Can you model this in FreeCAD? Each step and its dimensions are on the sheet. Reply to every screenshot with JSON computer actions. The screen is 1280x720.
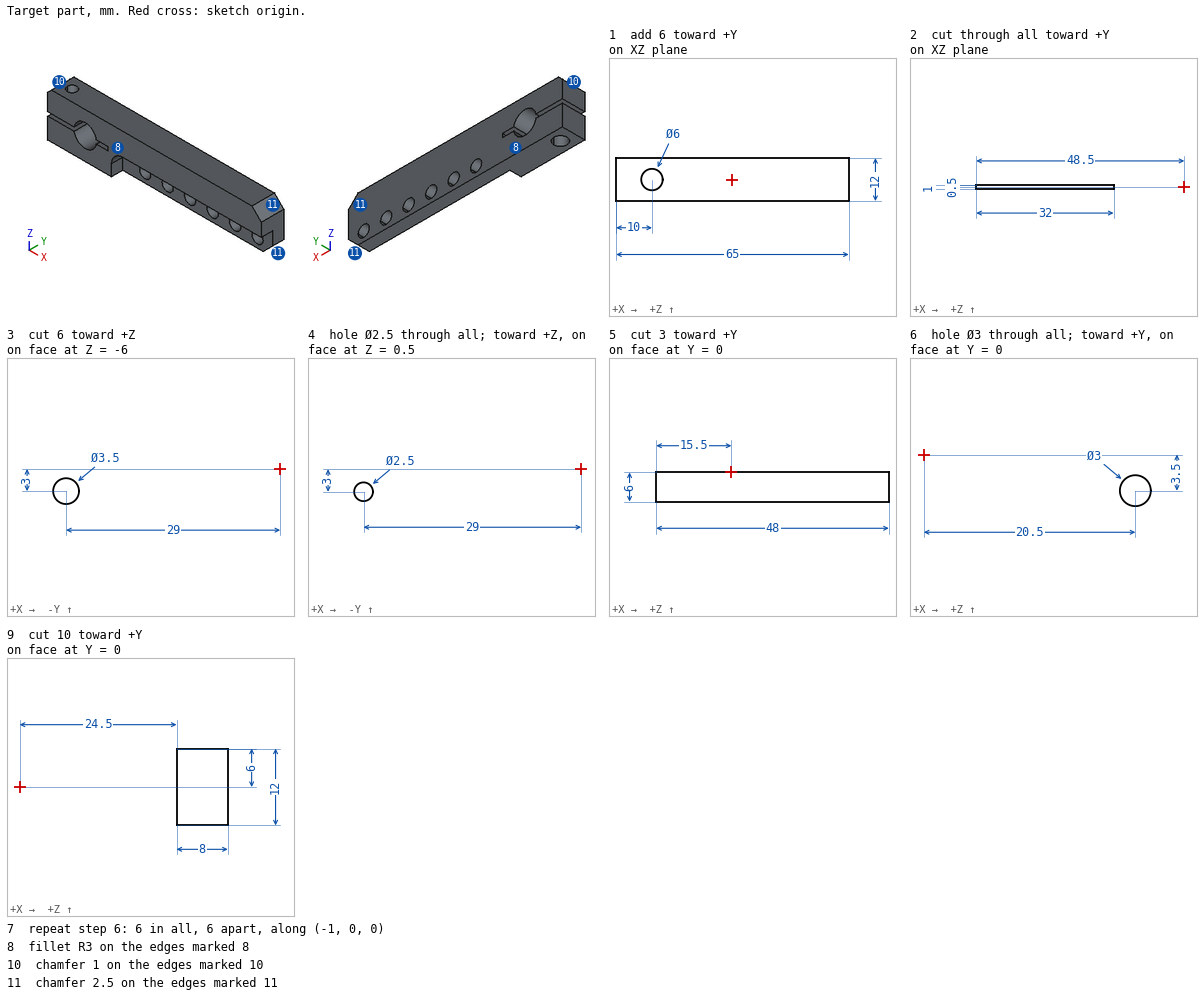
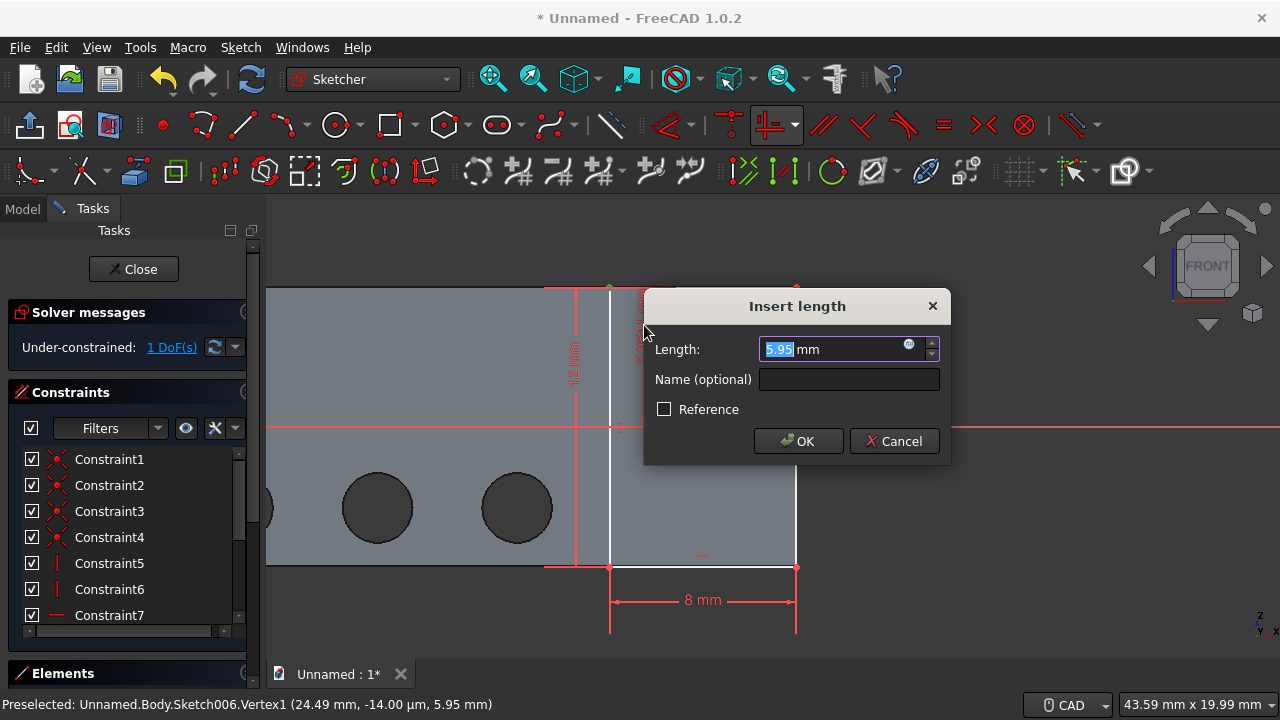
{"action": "type", "text": "6"}
{"action": "key", "text": "Return"}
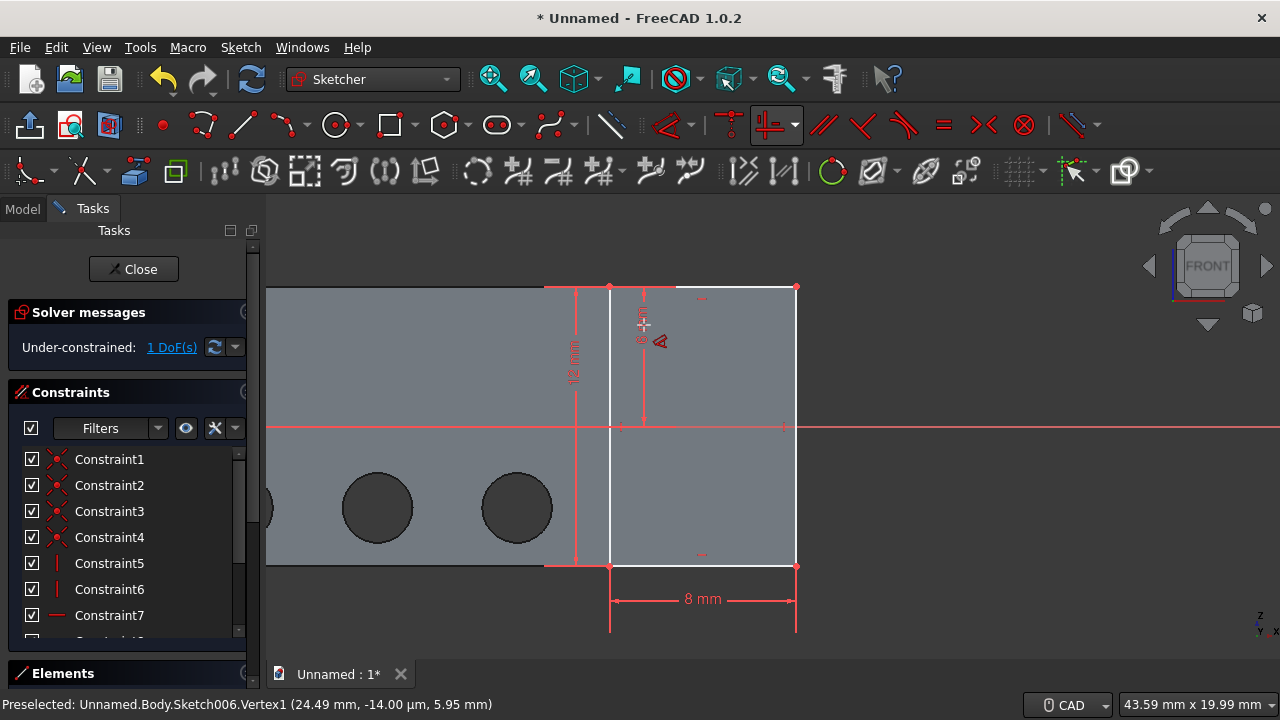
{"action": "left_click", "coordinate": [610, 287]}
{"action": "left_click", "coordinate": [452, 253]}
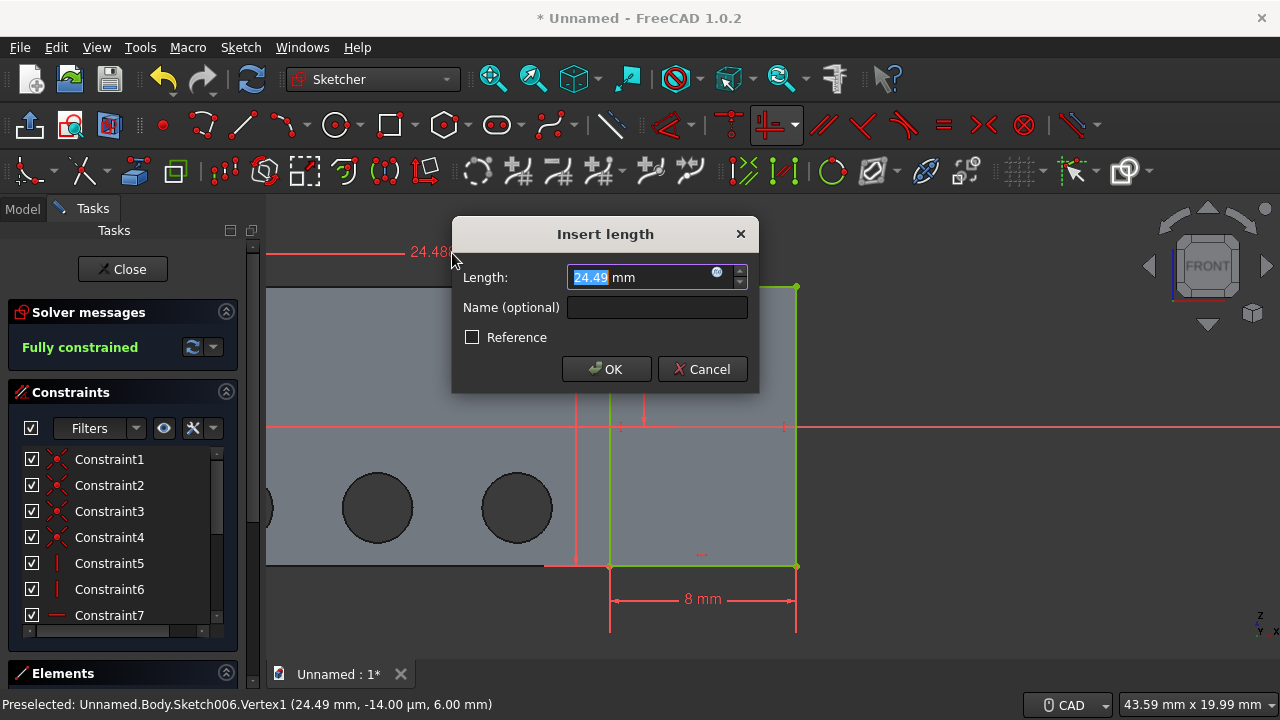
{"action": "type", "text": "24.5"}
{"action": "key", "text": "Return"}
{"action": "key", "text": "Escape"}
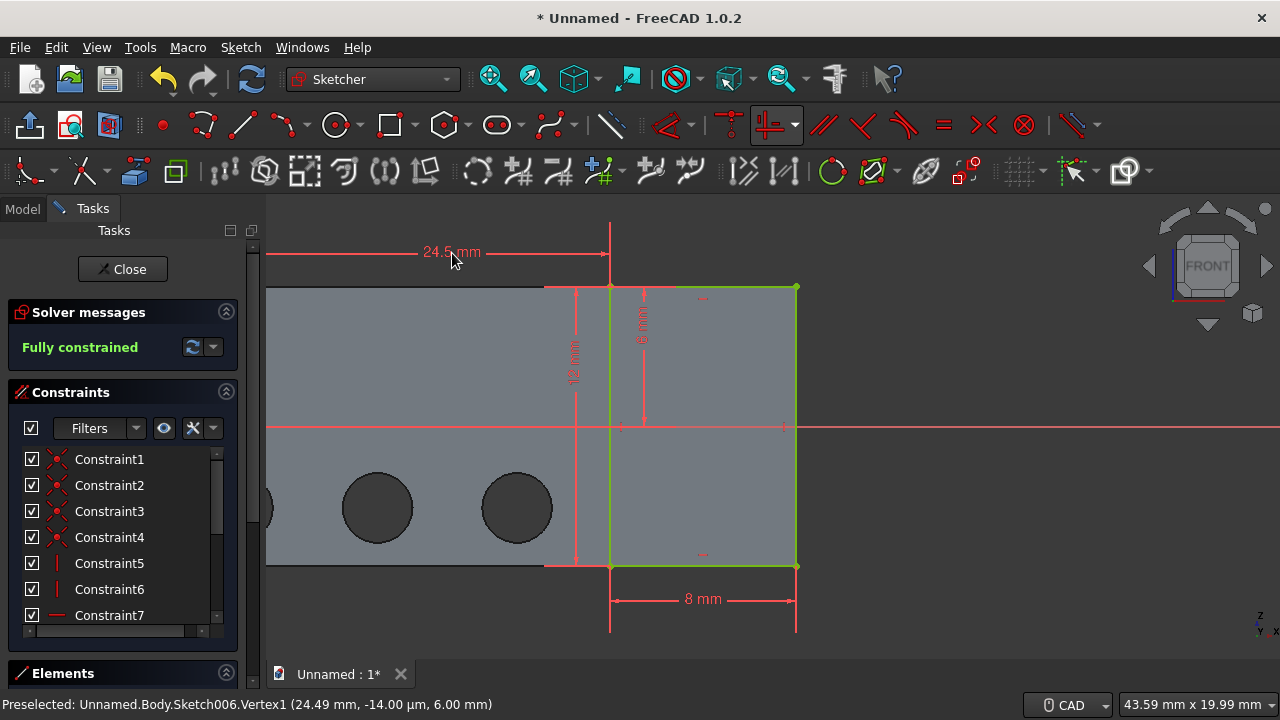
{"action": "left_click", "coordinate": [123, 269]}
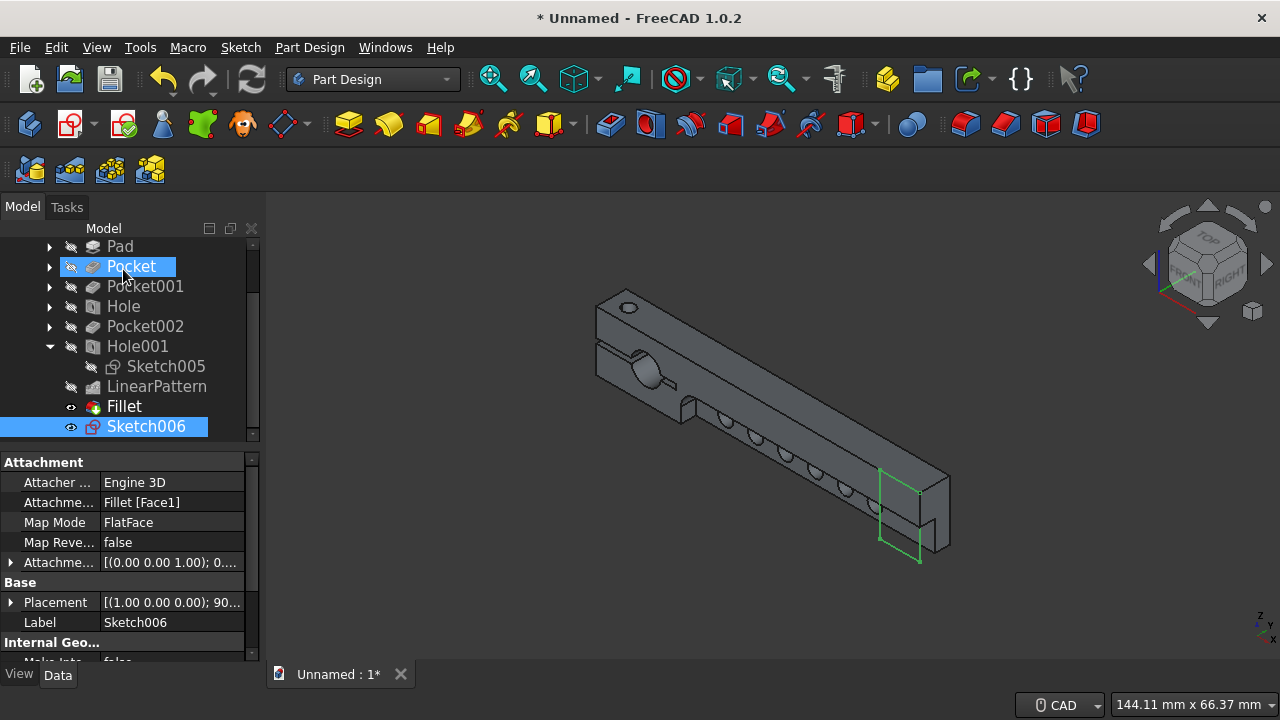
{"action": "left_click", "coordinate": [612, 124]}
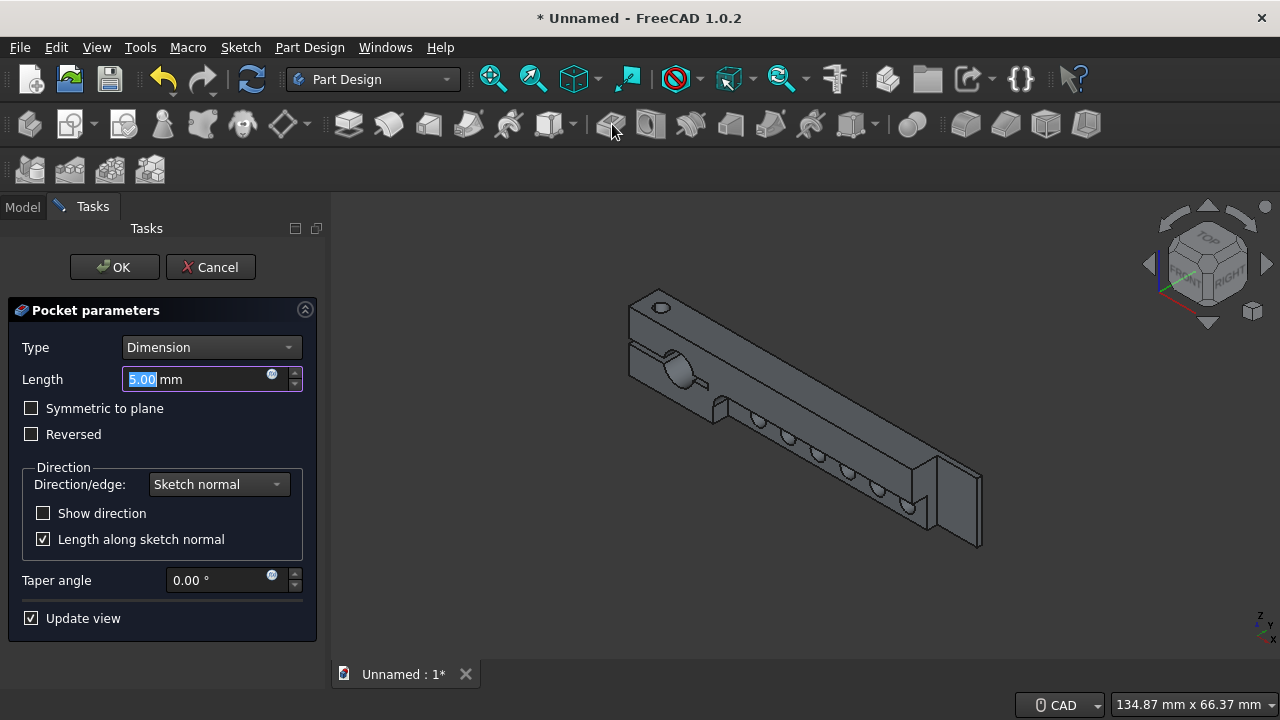
{"action": "type", "text": "10"}
{"action": "key", "text": "Tab"}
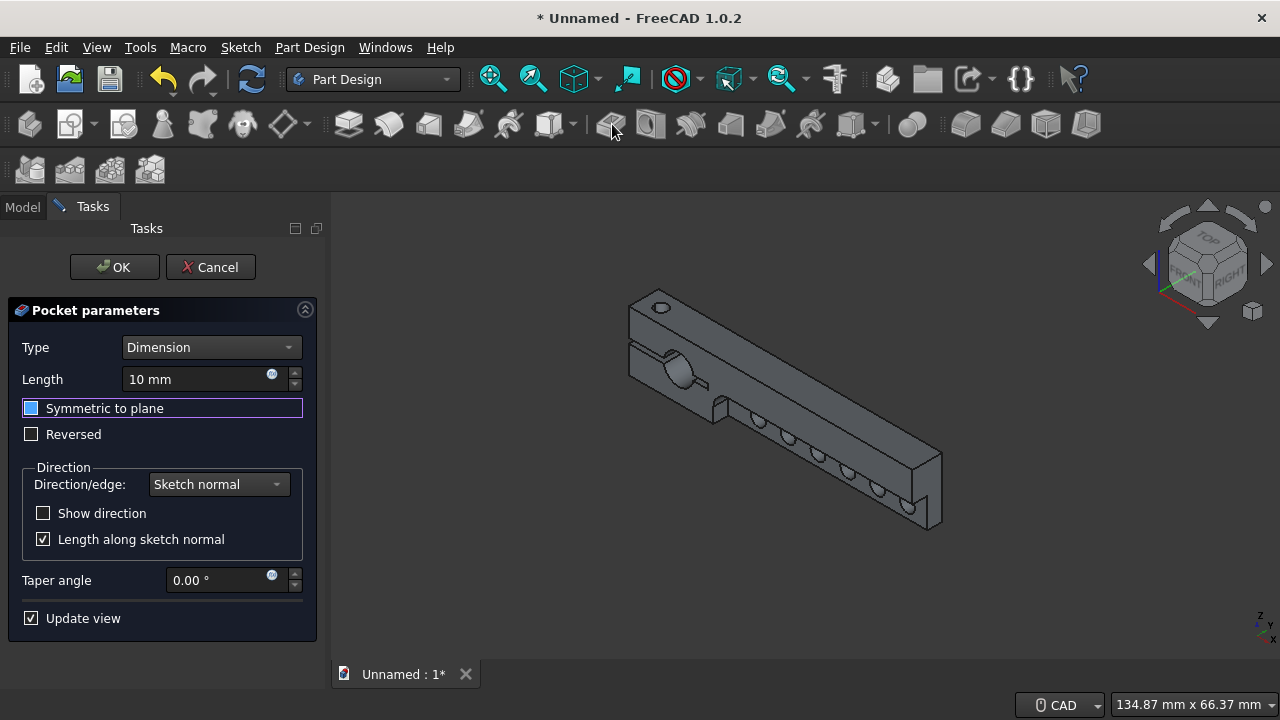
{"action": "left_click", "coordinate": [115, 267]}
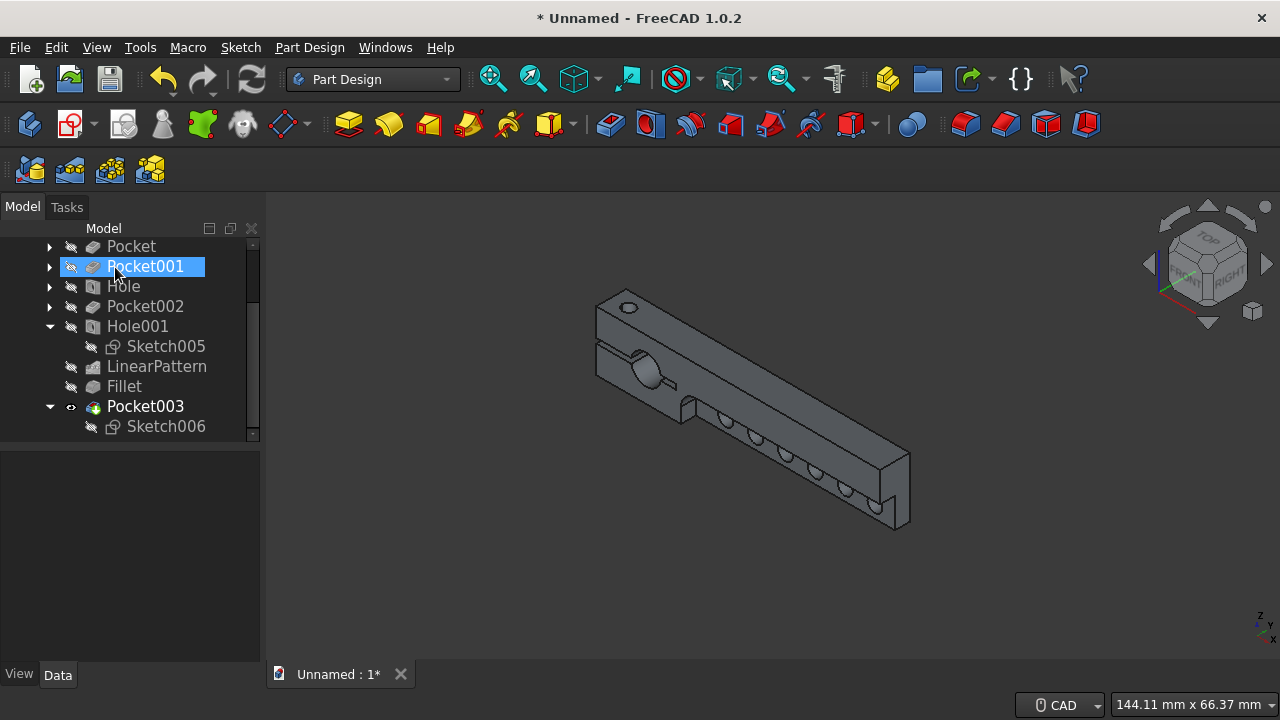
{"action": "key", "text": "2"}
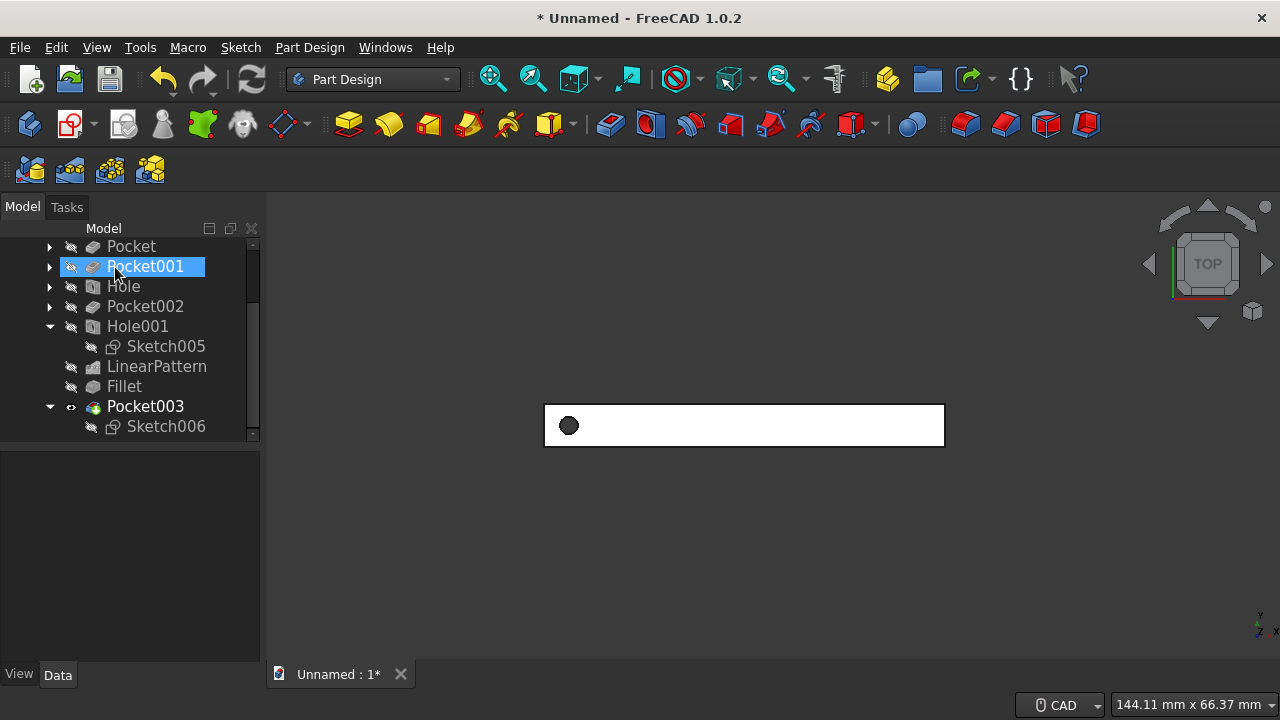
{"action": "left_click", "coordinate": [494, 80]}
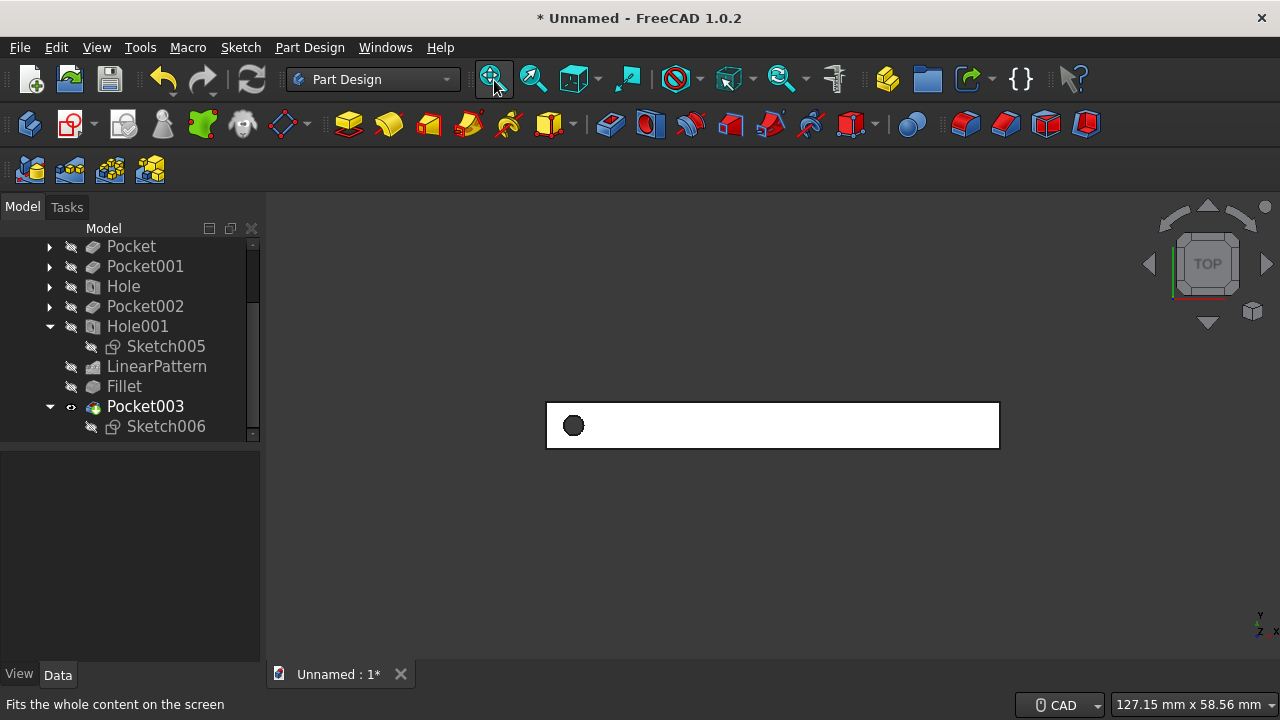
{"action": "left_click", "coordinate": [546, 424]}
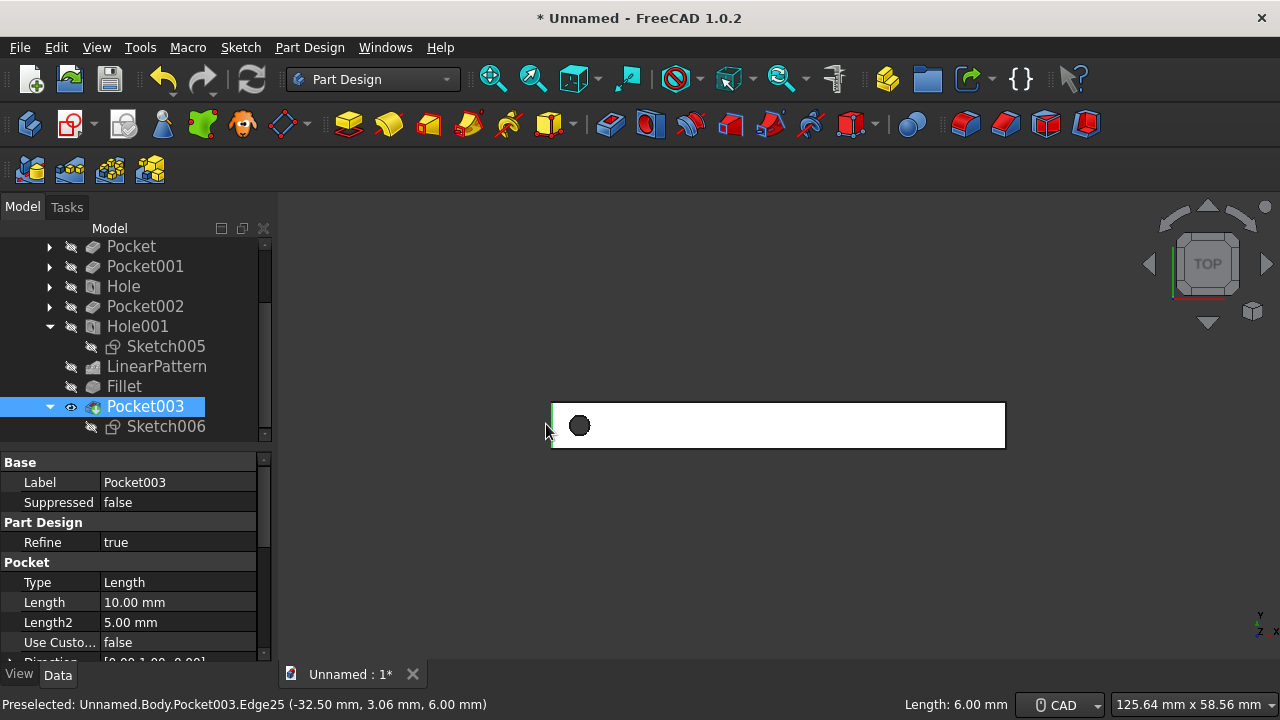
{"action": "left_click", "coordinate": [1006, 124]}